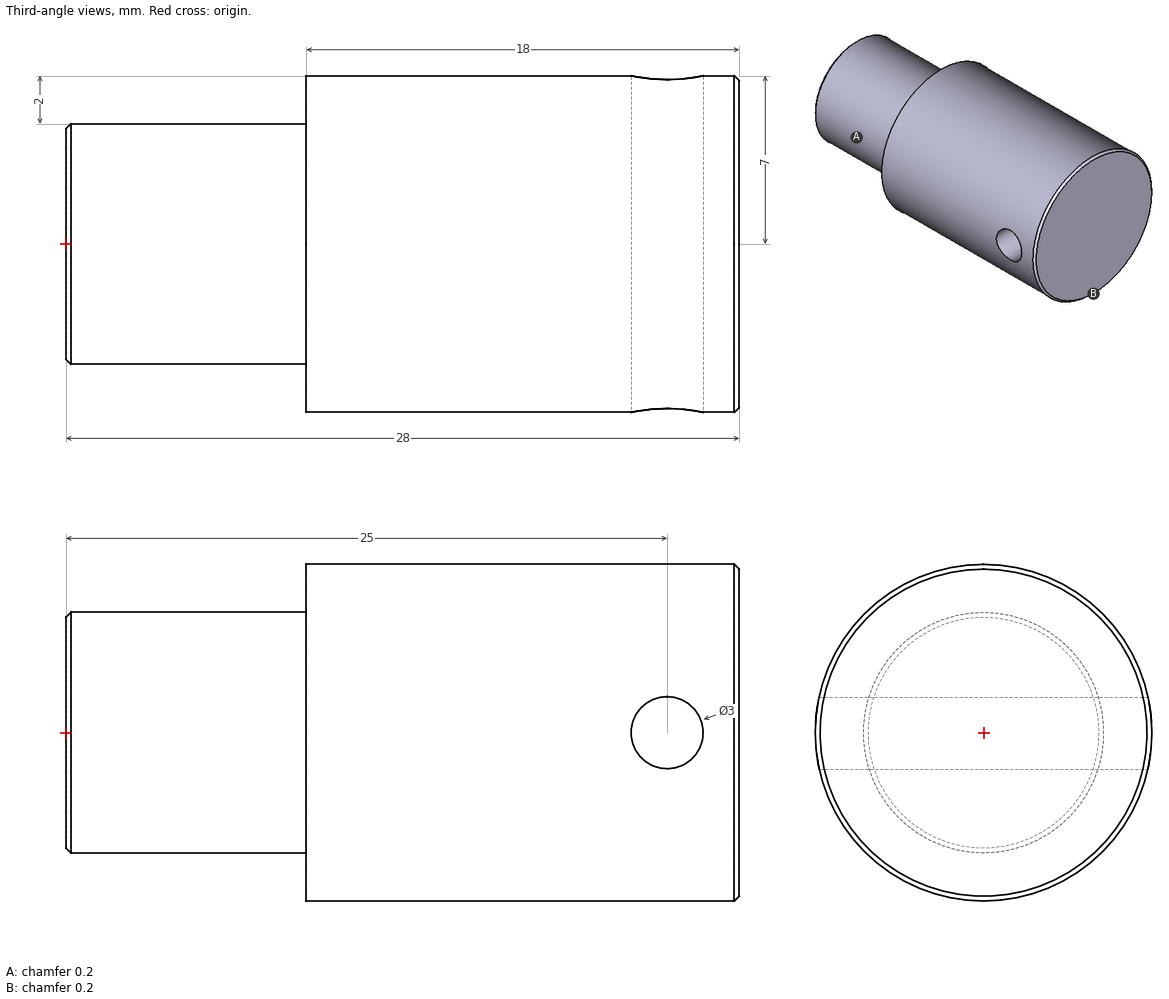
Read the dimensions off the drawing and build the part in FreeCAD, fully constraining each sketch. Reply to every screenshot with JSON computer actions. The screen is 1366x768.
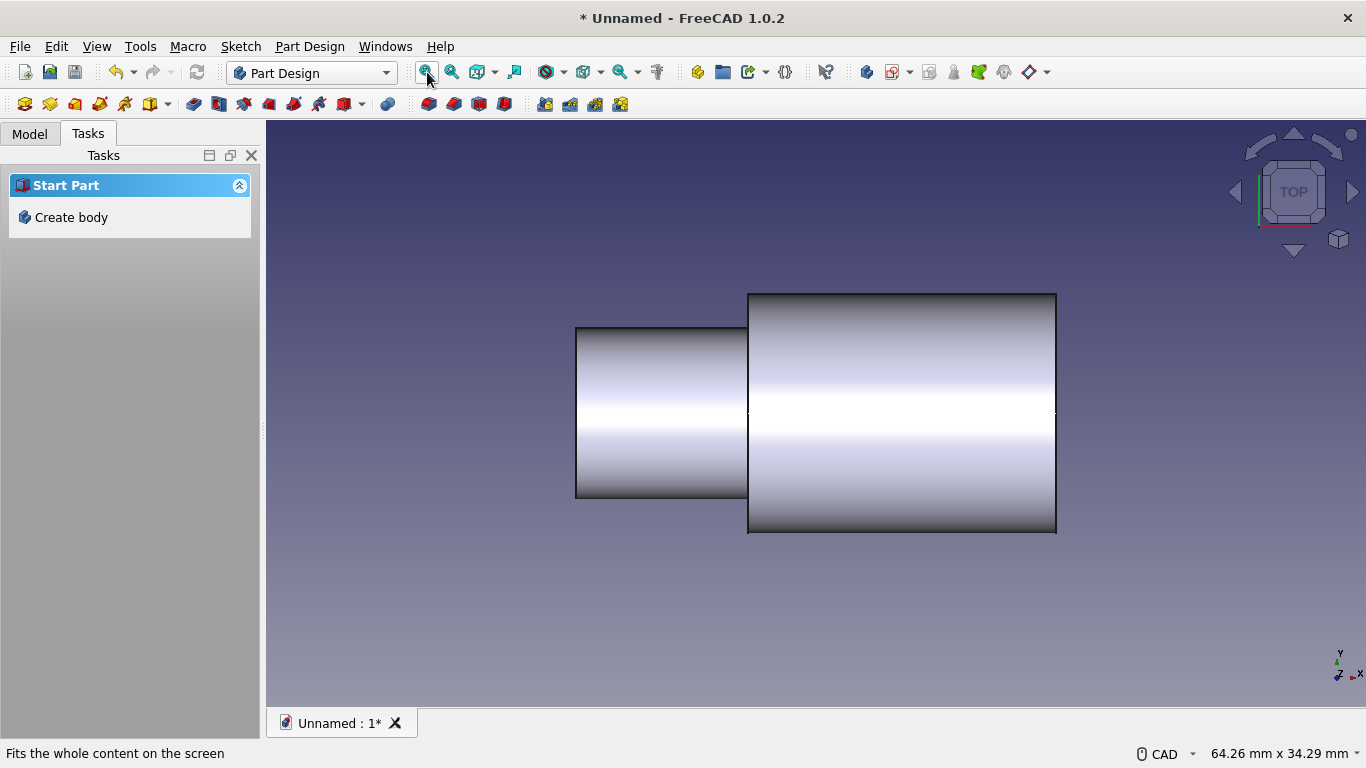
{"action": "left_click", "coordinate": [576, 482]}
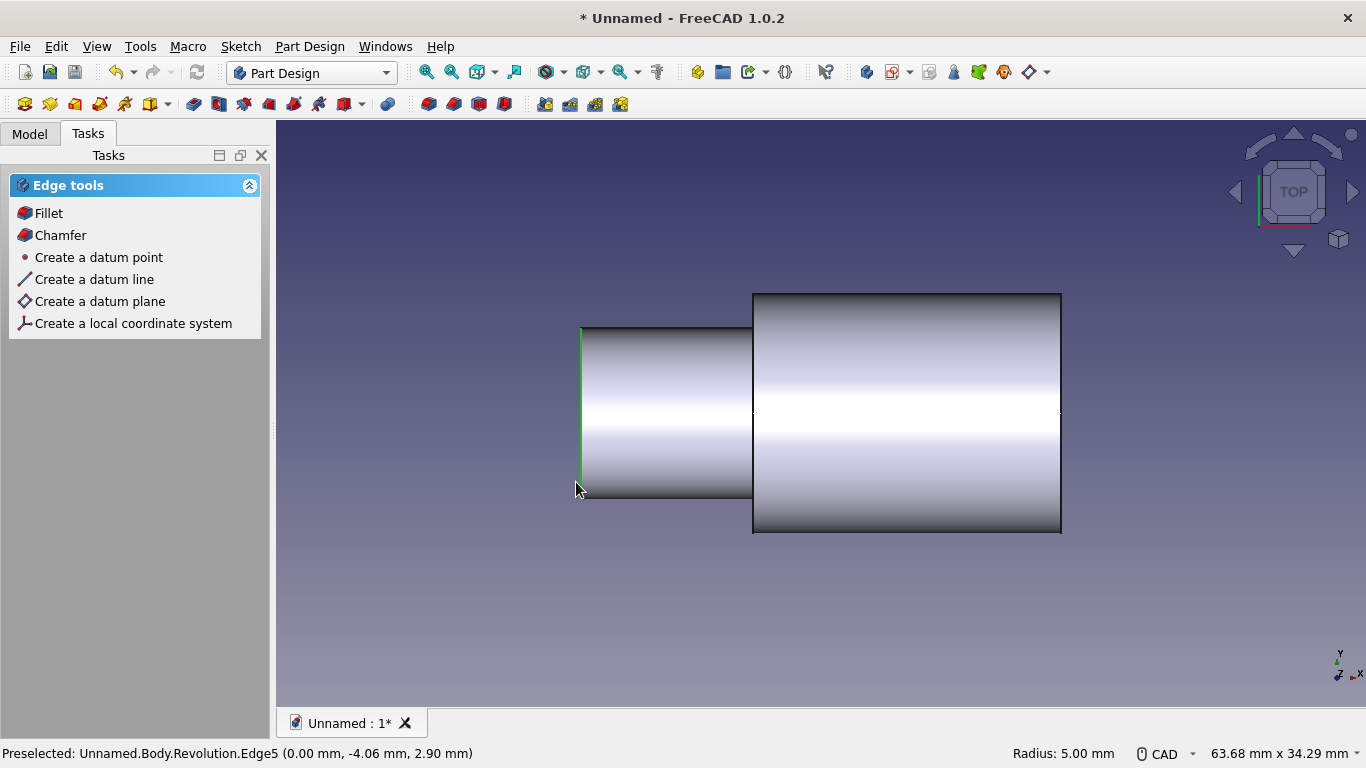
{"action": "left_click", "coordinate": [454, 104]}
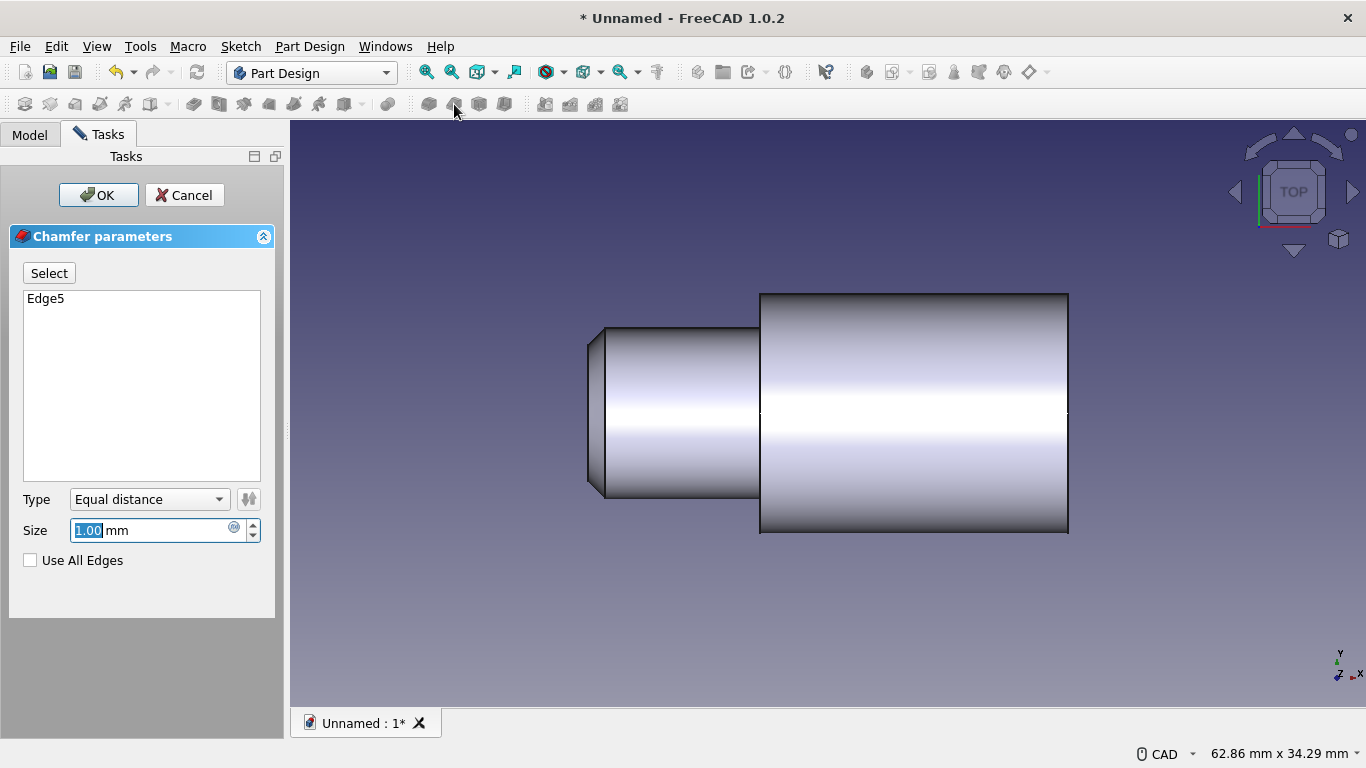
{"action": "type", "text": "0.2"}
{"action": "key", "text": "Tab"}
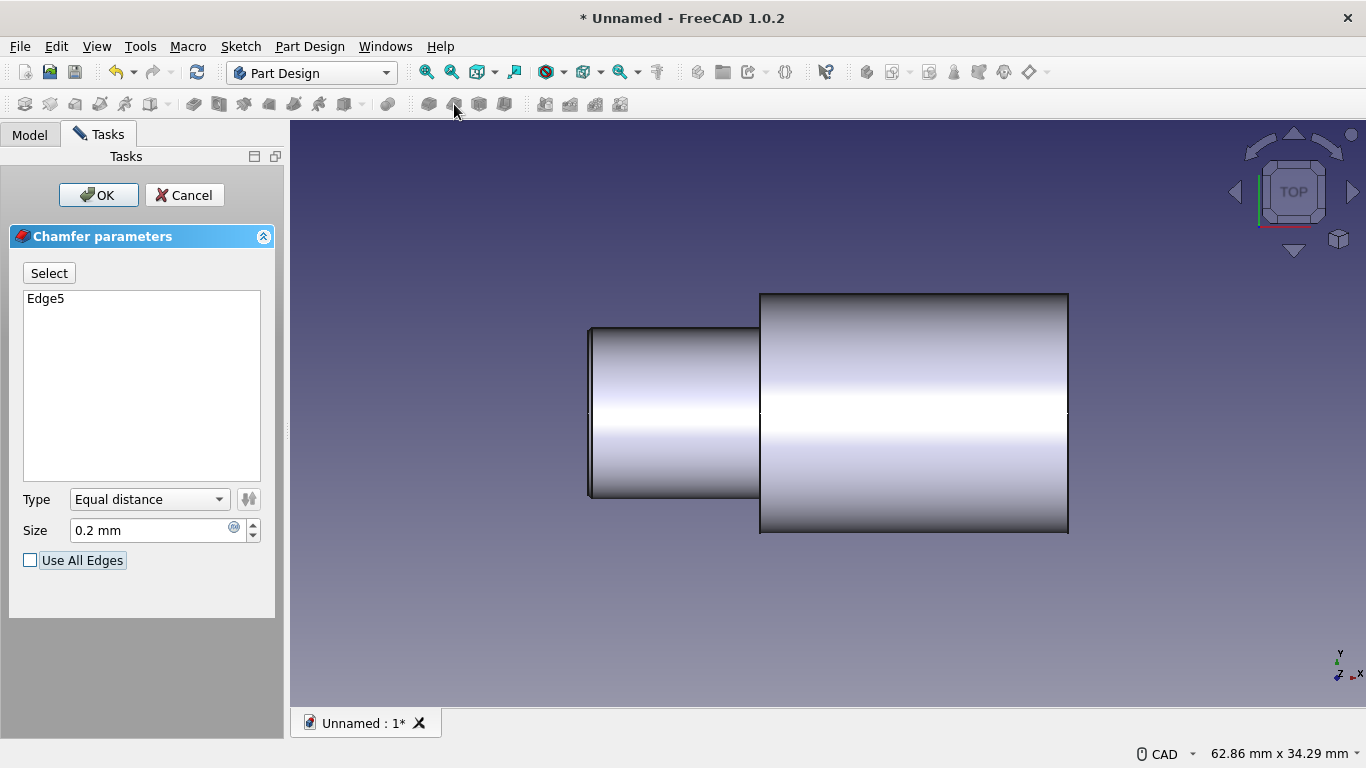
{"action": "left_click", "coordinate": [99, 195]}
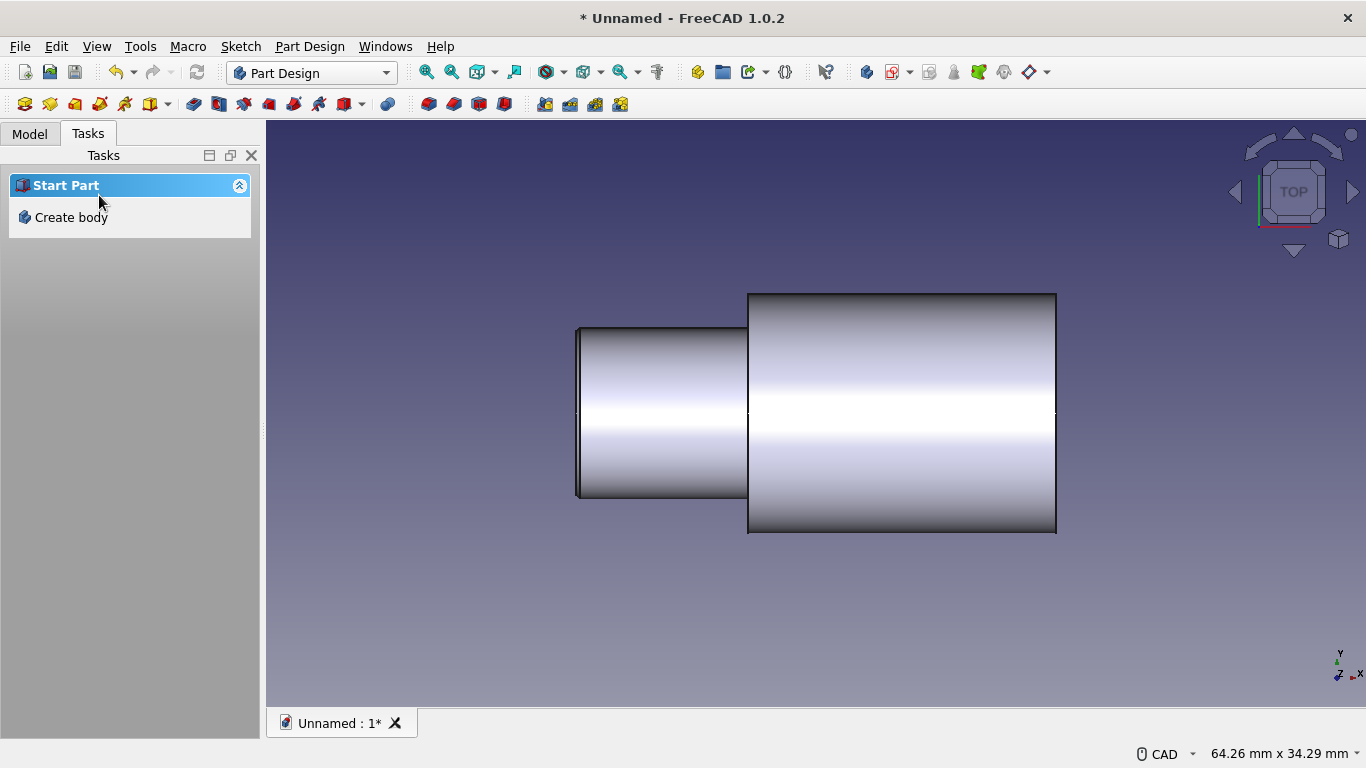
{"action": "left_click", "coordinate": [427, 72]}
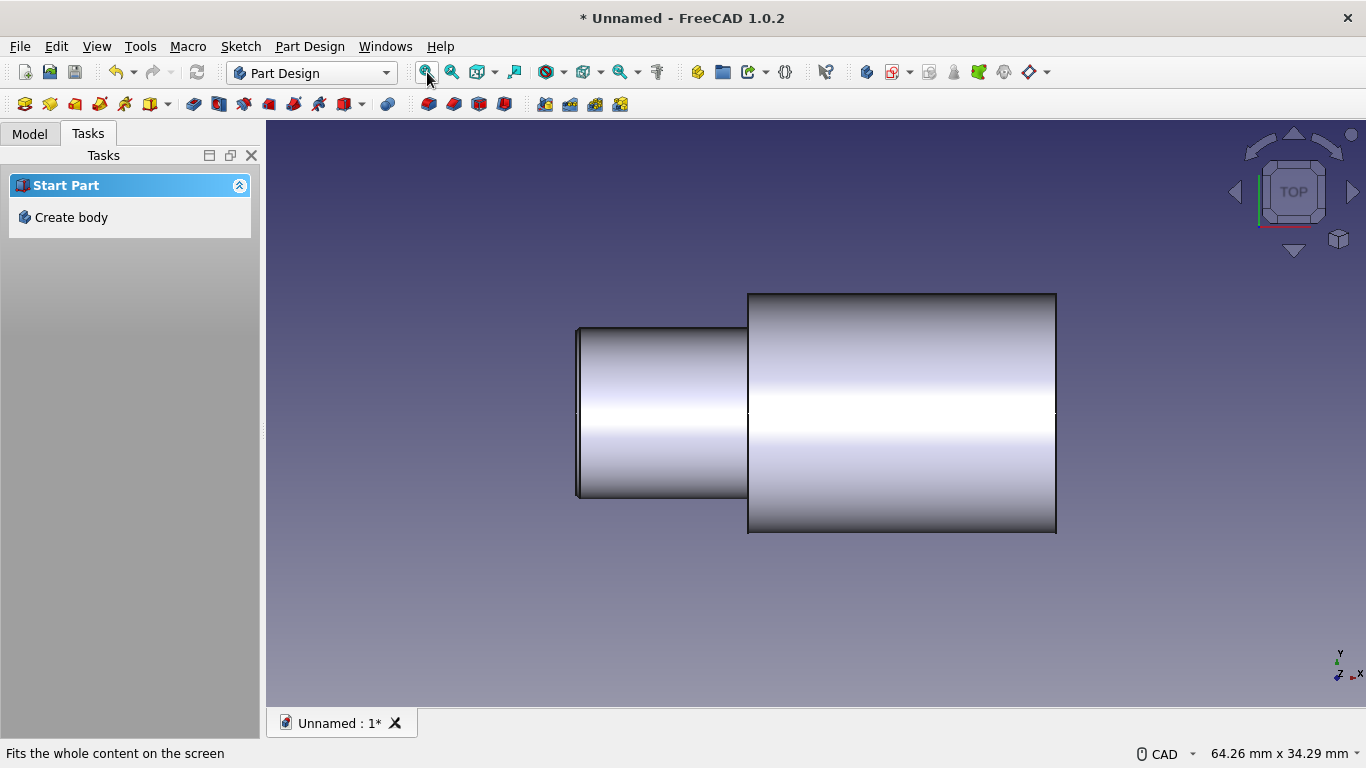
{"action": "left_click", "coordinate": [892, 72]}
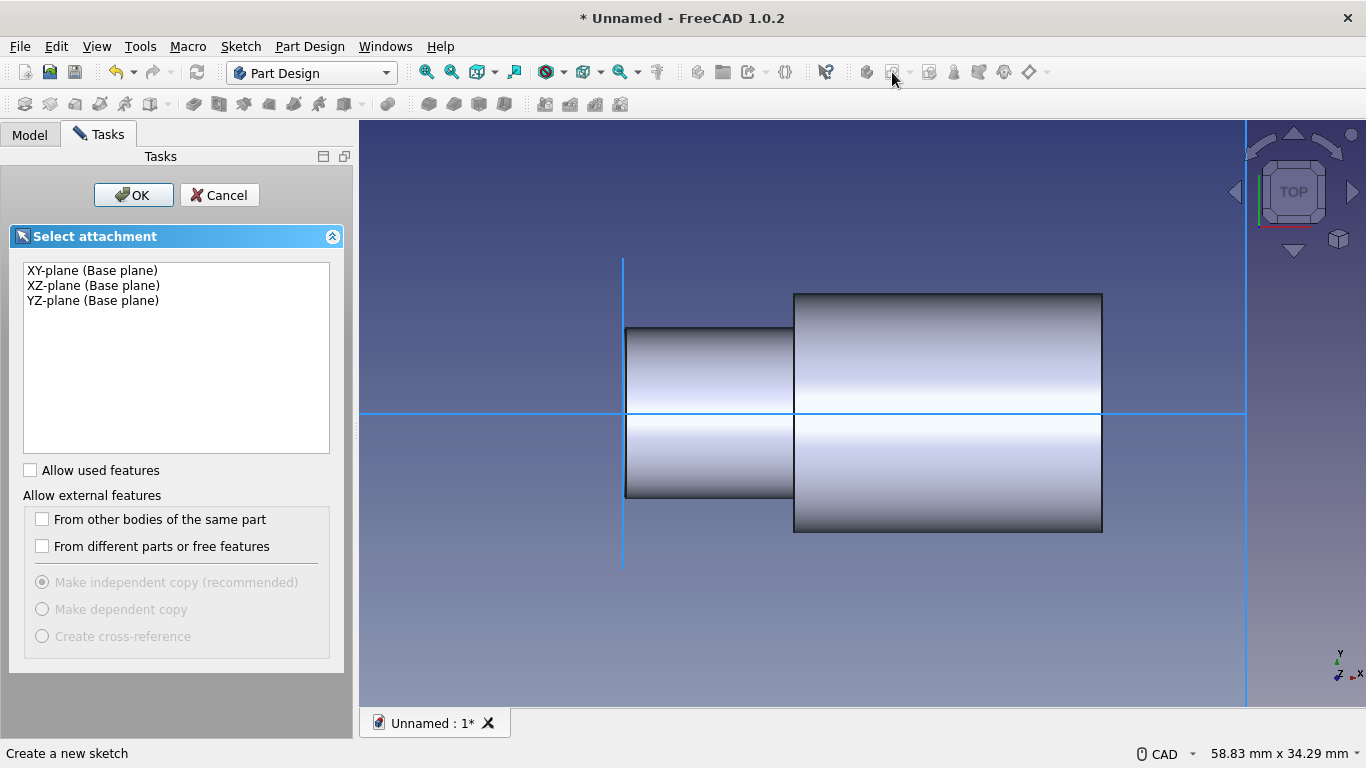
{"action": "left_click", "coordinate": [84, 286]}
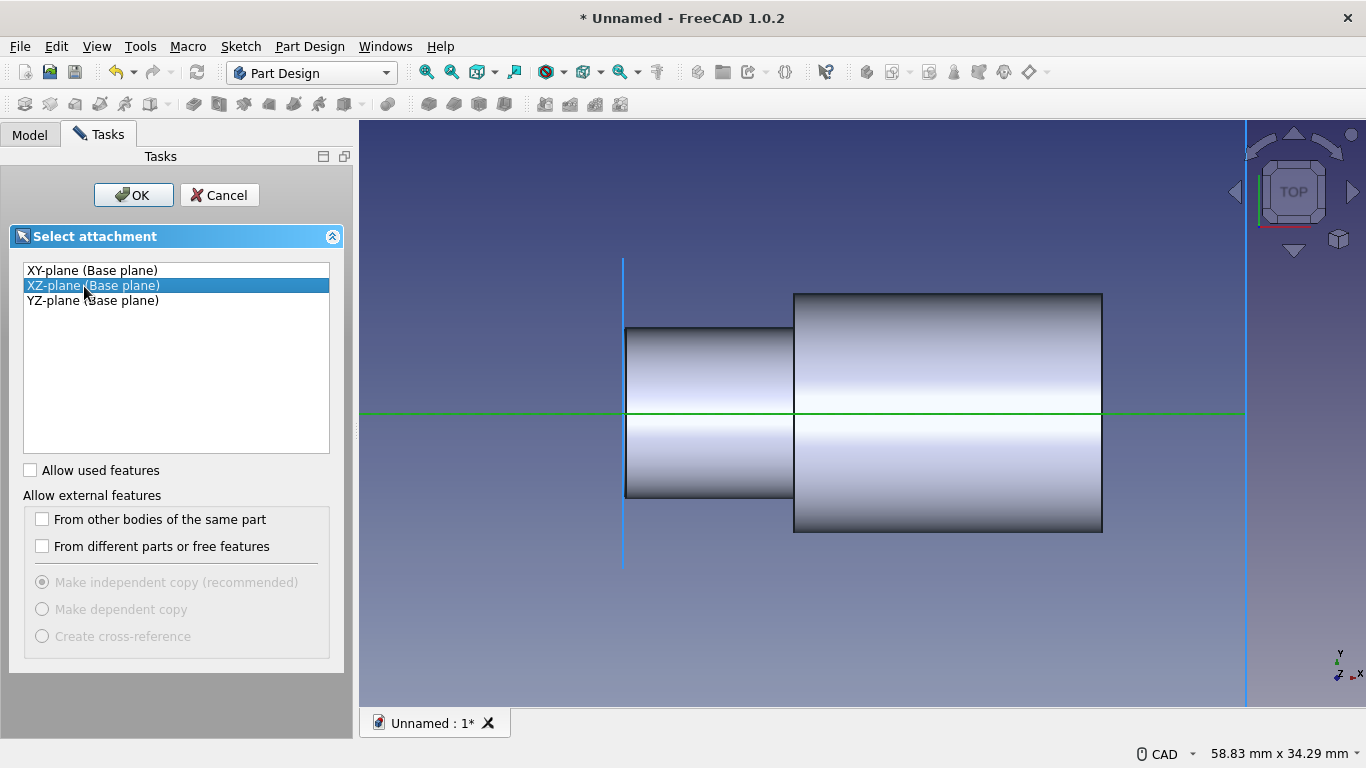
{"action": "left_click", "coordinate": [134, 195]}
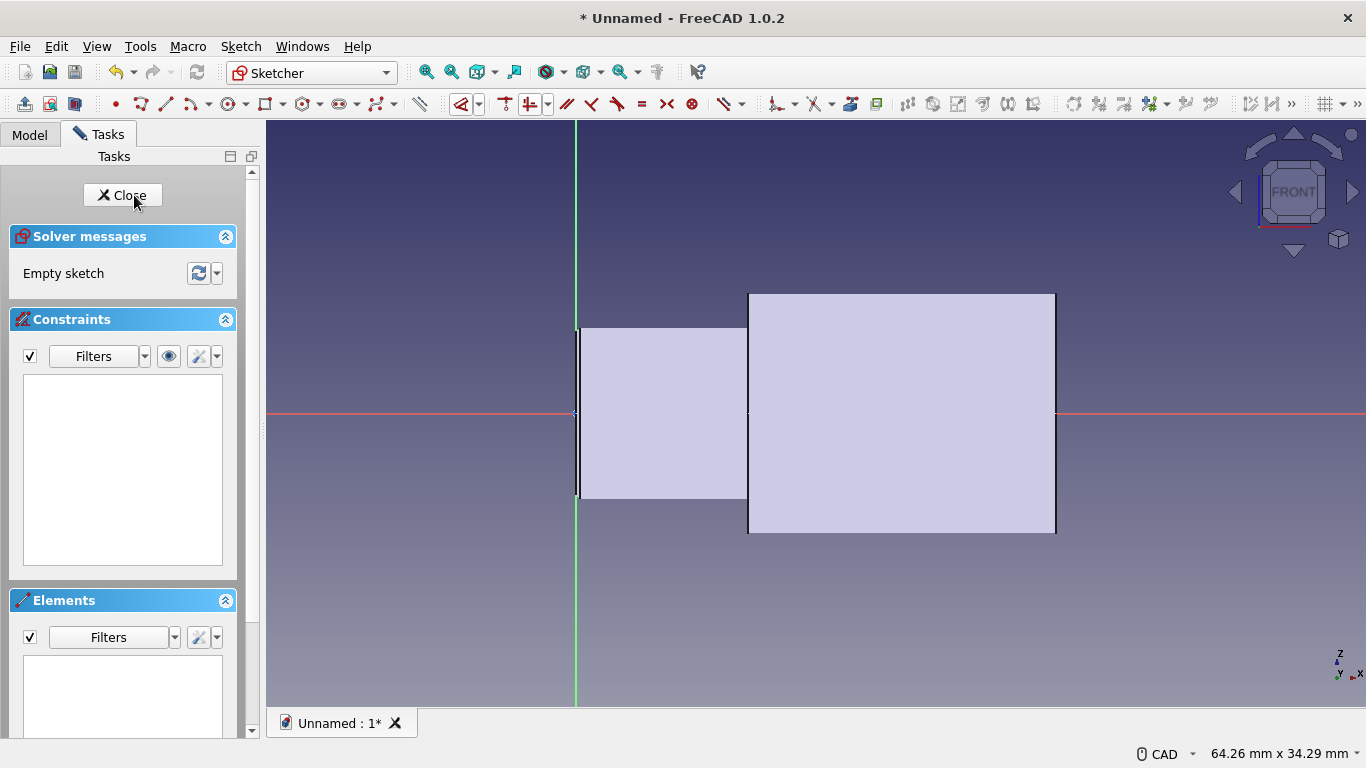
{"action": "key", "text": "q s"}